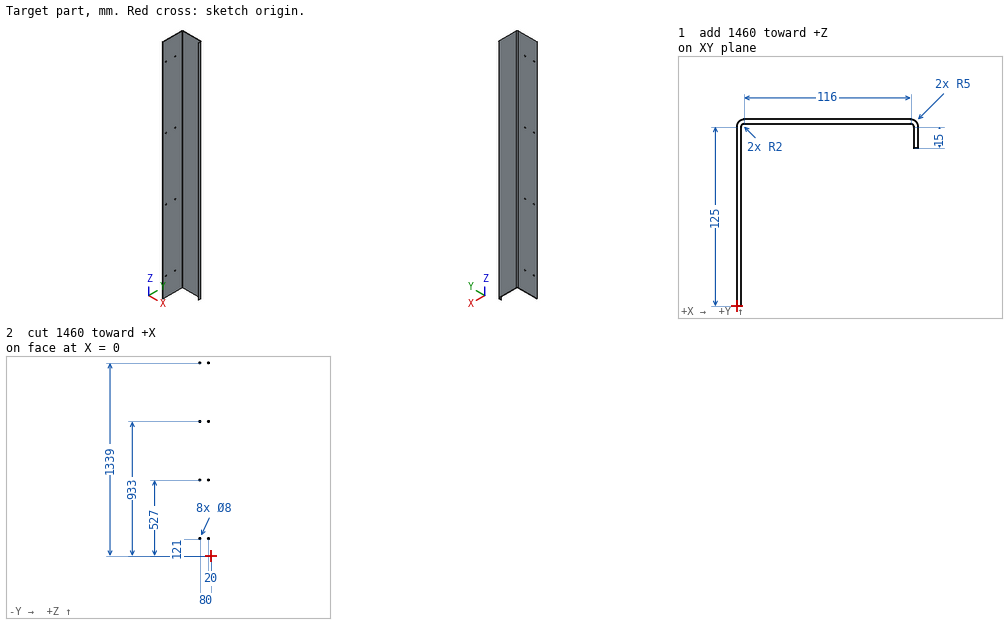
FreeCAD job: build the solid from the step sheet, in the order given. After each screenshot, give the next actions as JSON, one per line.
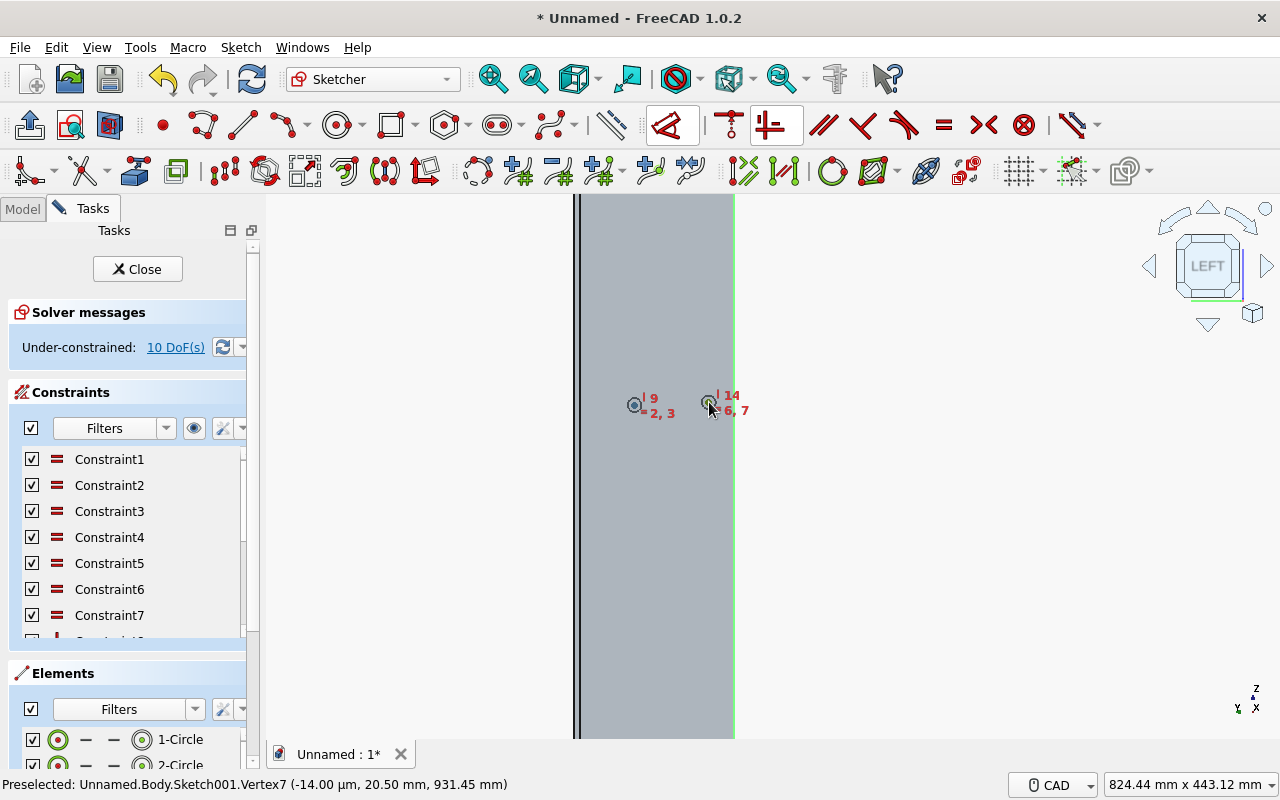
{"action": "key", "text": "h"}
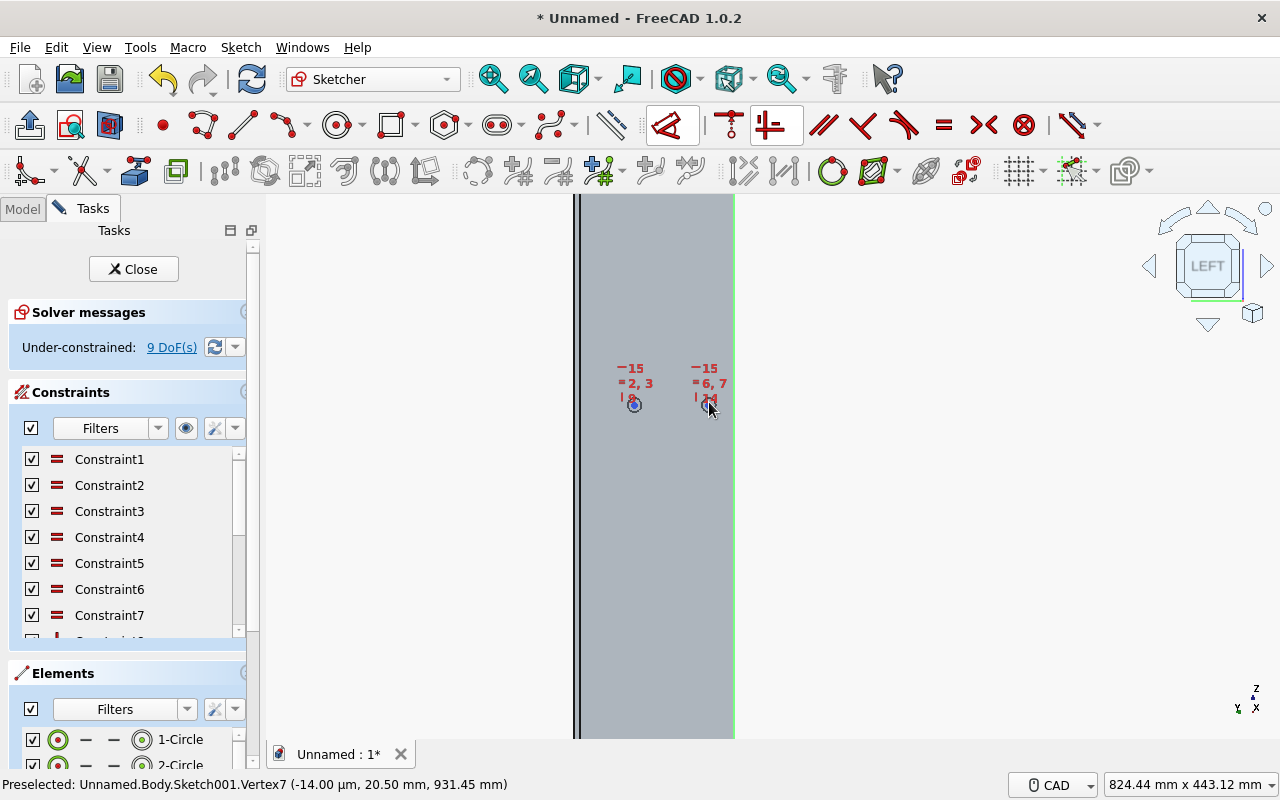
{"action": "scroll", "coordinate": [710, 402], "scroll_direction": "down", "scroll_amount": 8}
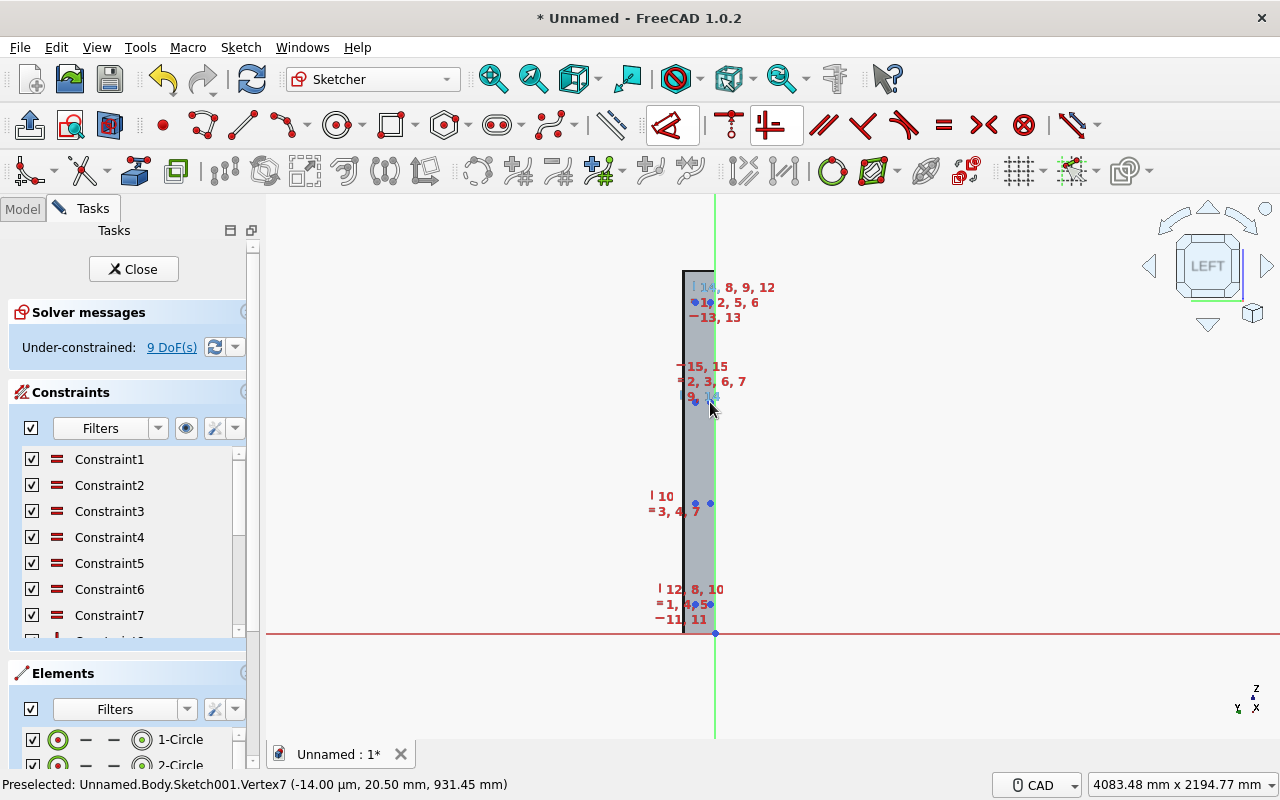
{"action": "left_click", "coordinate": [710, 604]}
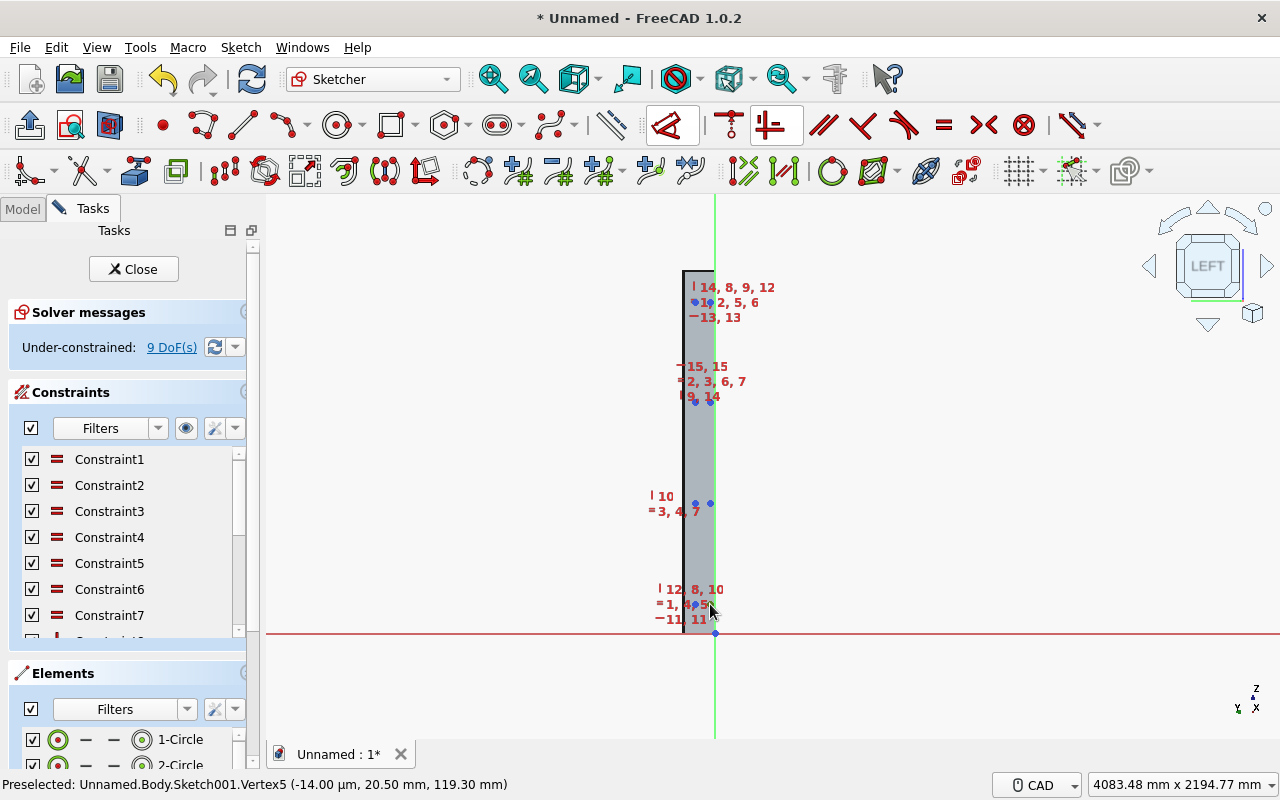
{"action": "left_click", "coordinate": [710, 503]}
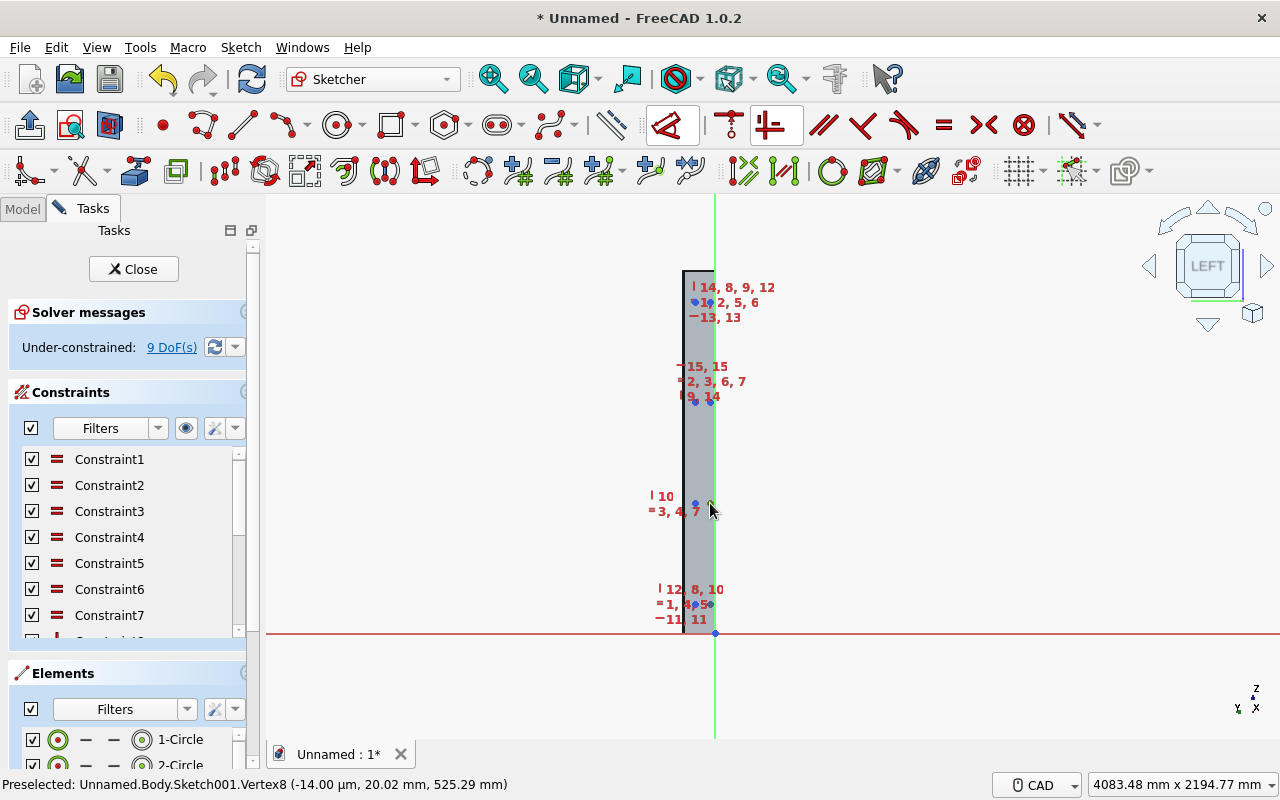
{"action": "key", "text": "v"}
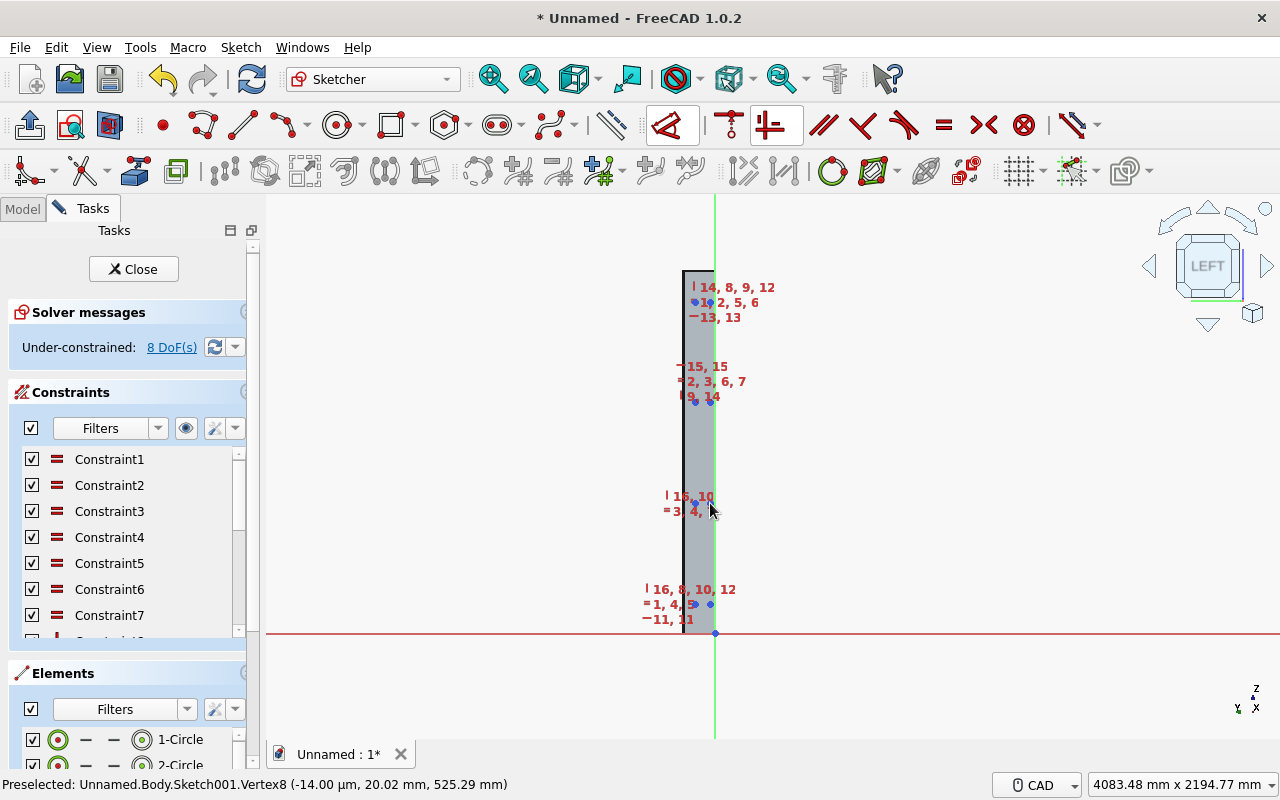
{"action": "scroll", "coordinate": [695, 504], "scroll_direction": "up", "scroll_amount": 4}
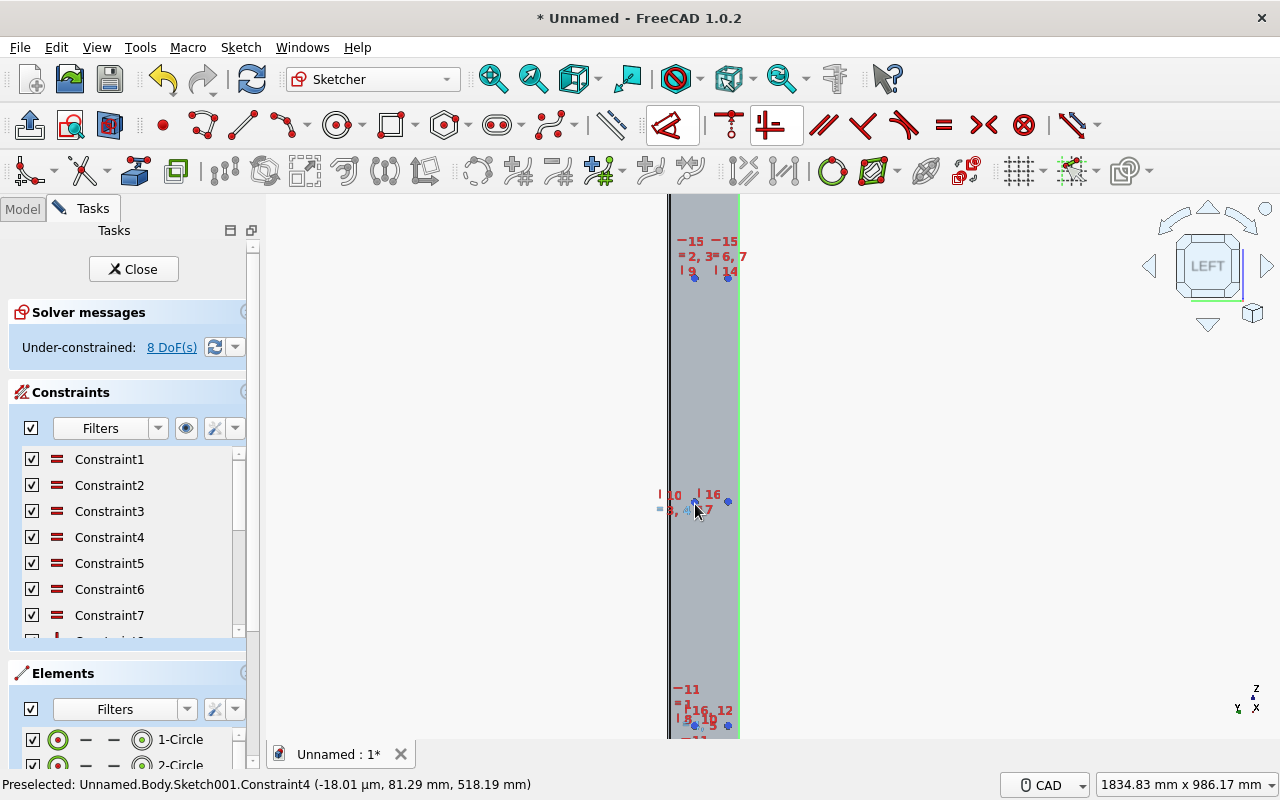
{"action": "scroll", "coordinate": [695, 502], "scroll_direction": "up", "scroll_amount": 4}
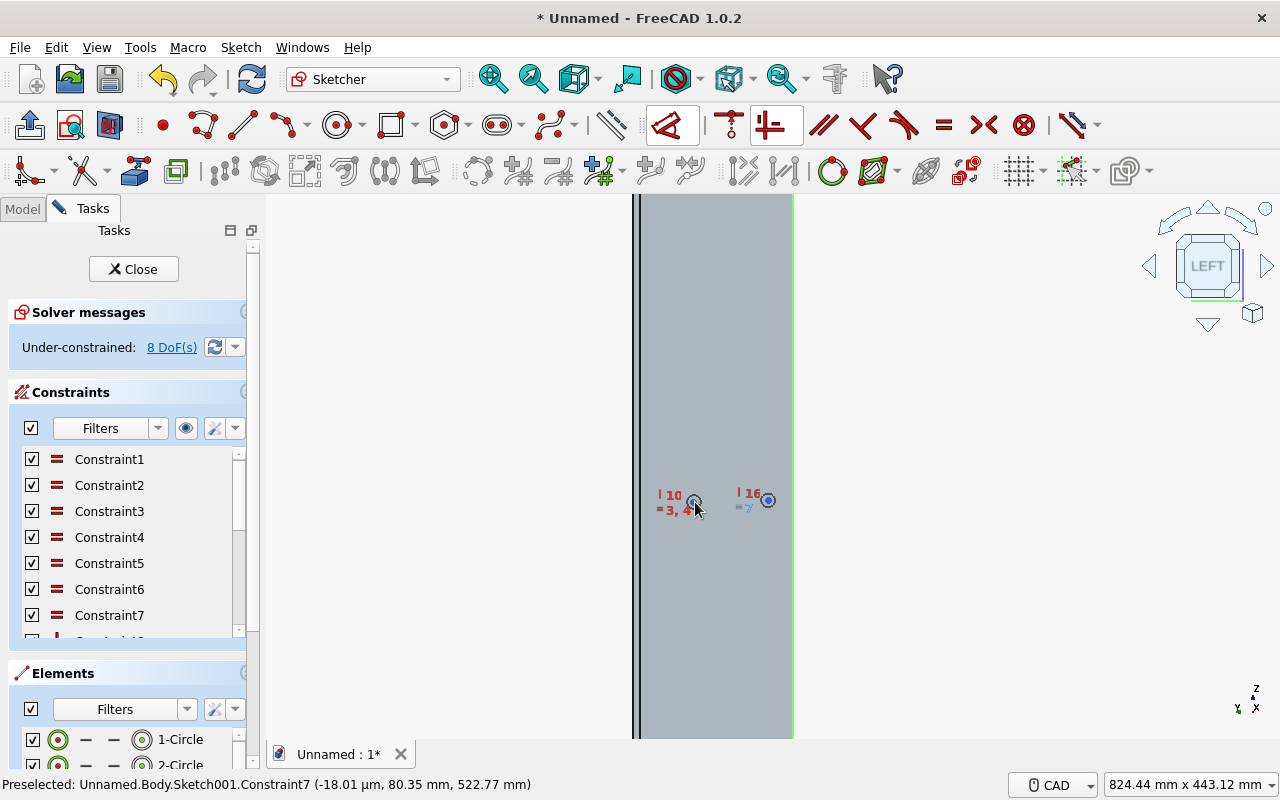
{"action": "left_click", "coordinate": [694, 502]}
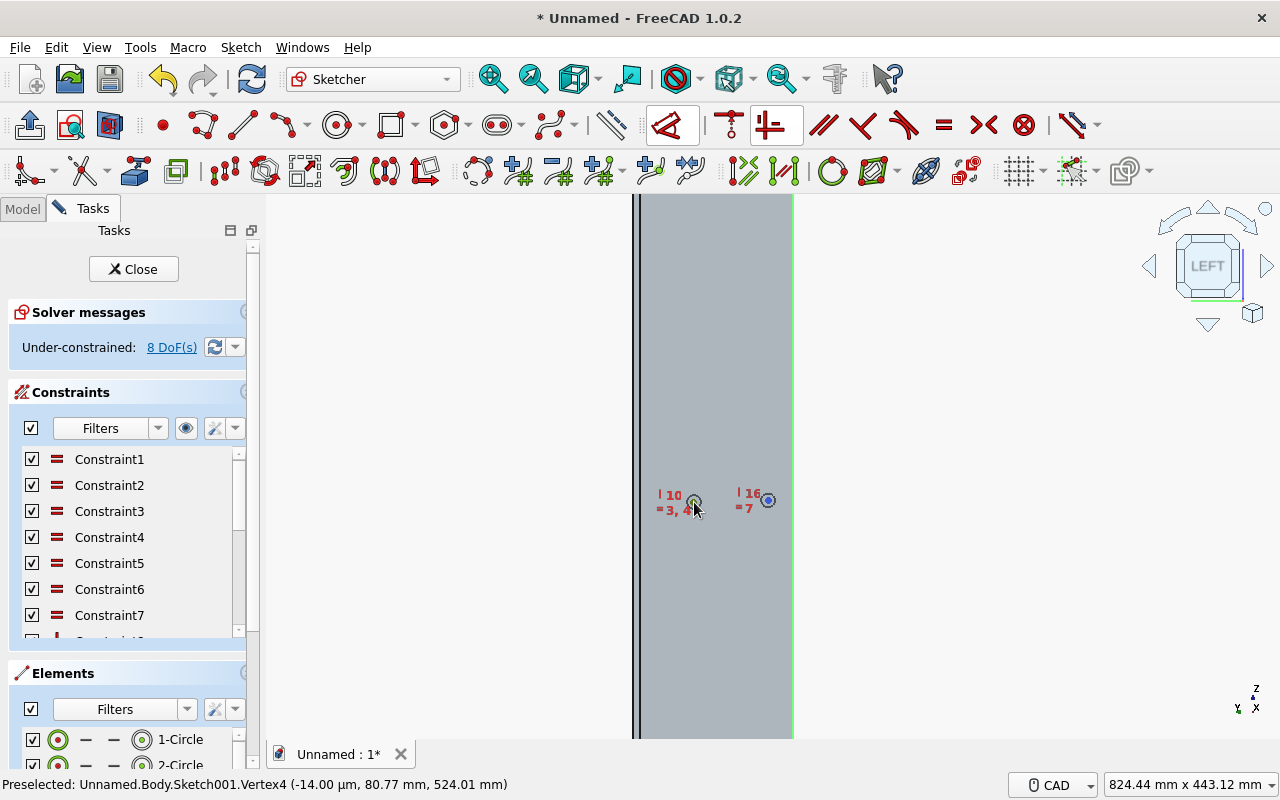
{"action": "scroll", "coordinate": [695, 503], "scroll_direction": "down", "scroll_amount": 8}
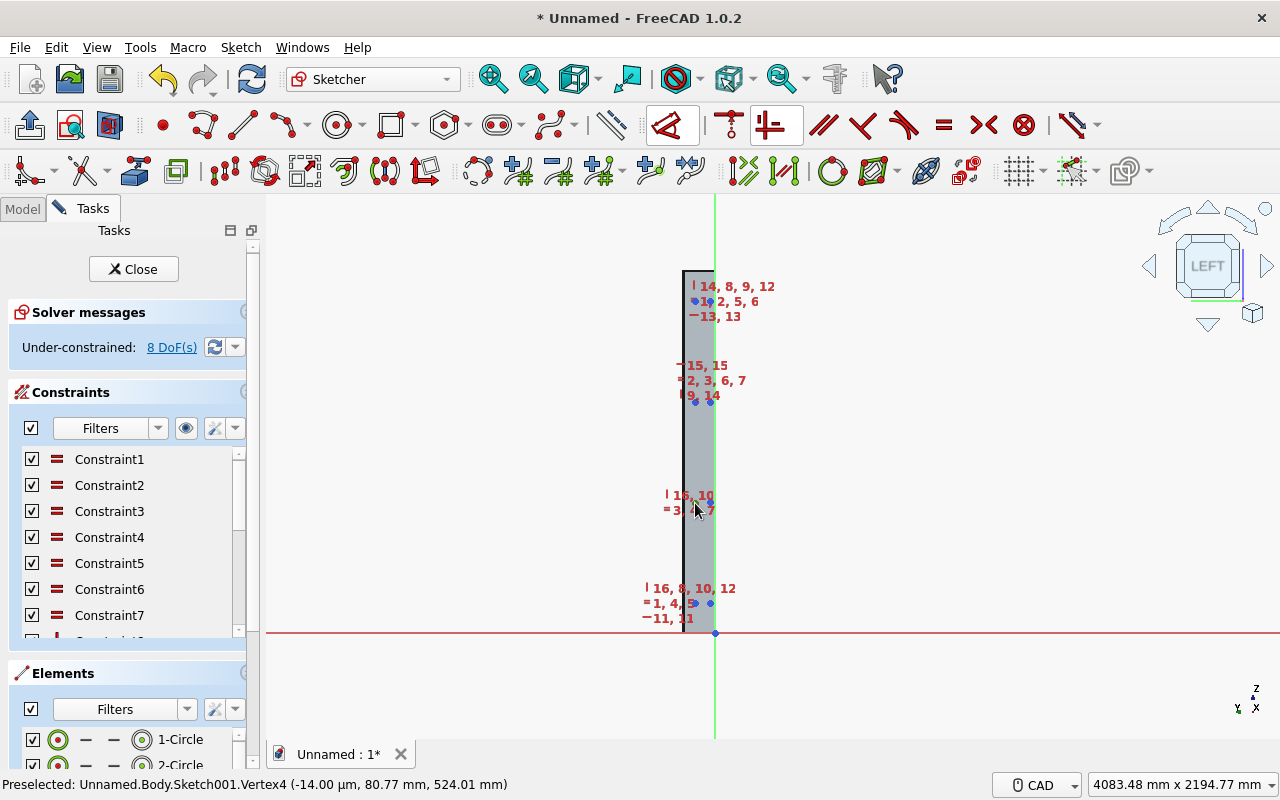
{"action": "scroll", "coordinate": [710, 503], "scroll_direction": "up", "scroll_amount": 4}